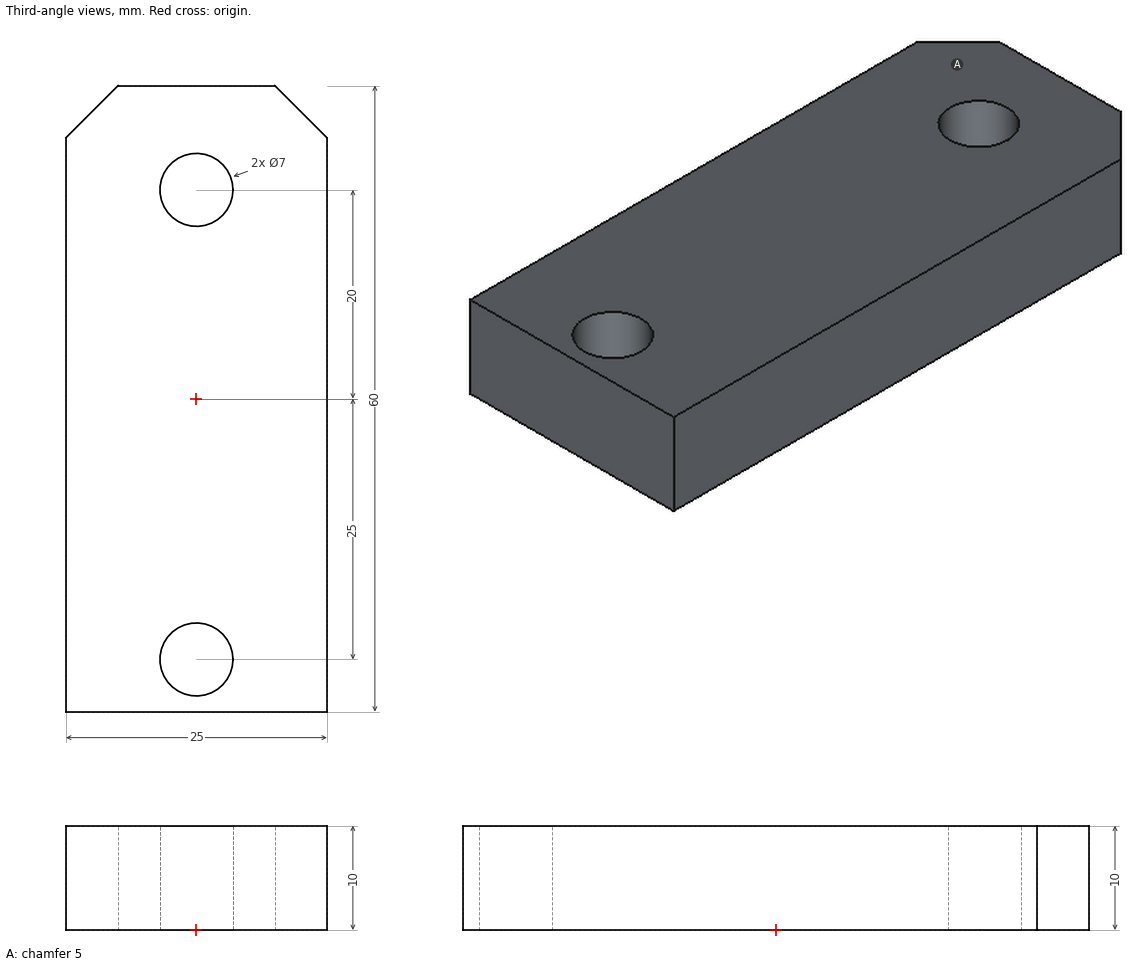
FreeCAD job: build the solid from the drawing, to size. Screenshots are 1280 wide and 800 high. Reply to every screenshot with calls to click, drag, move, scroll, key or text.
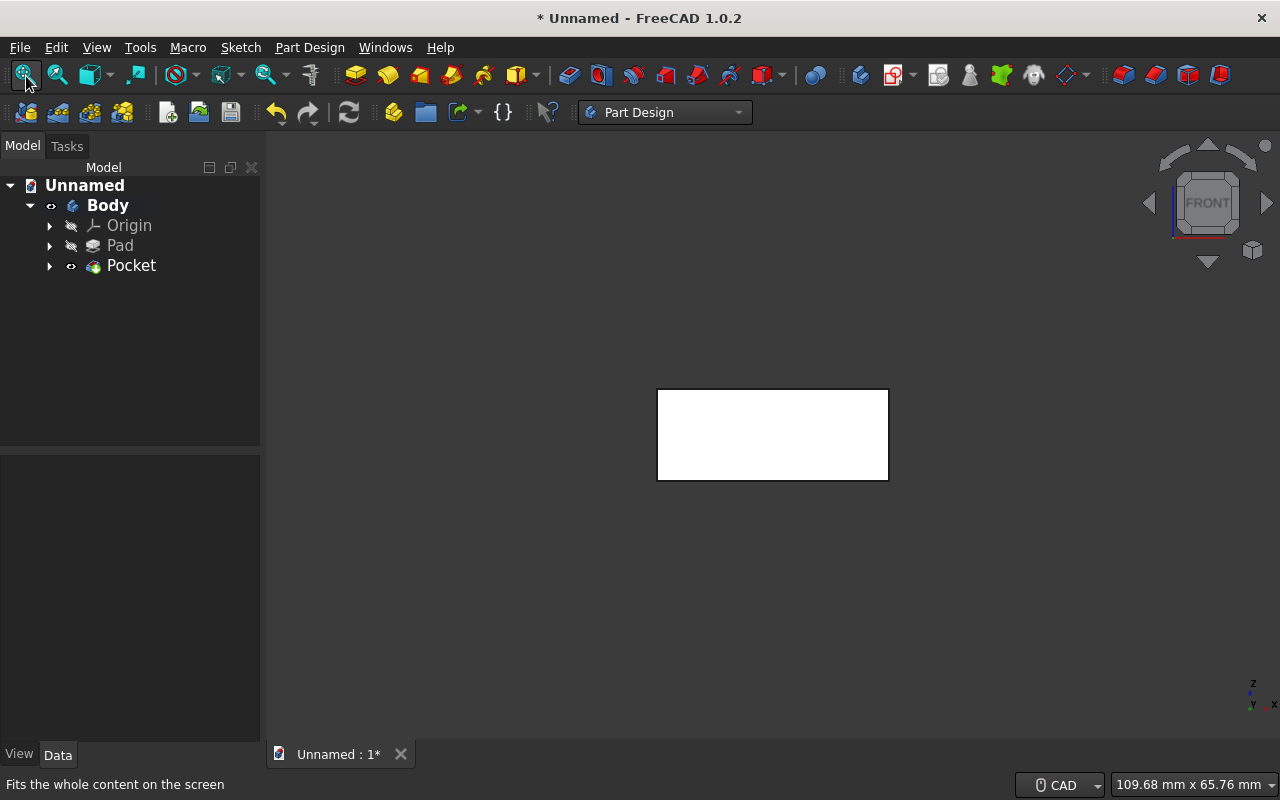
key(3)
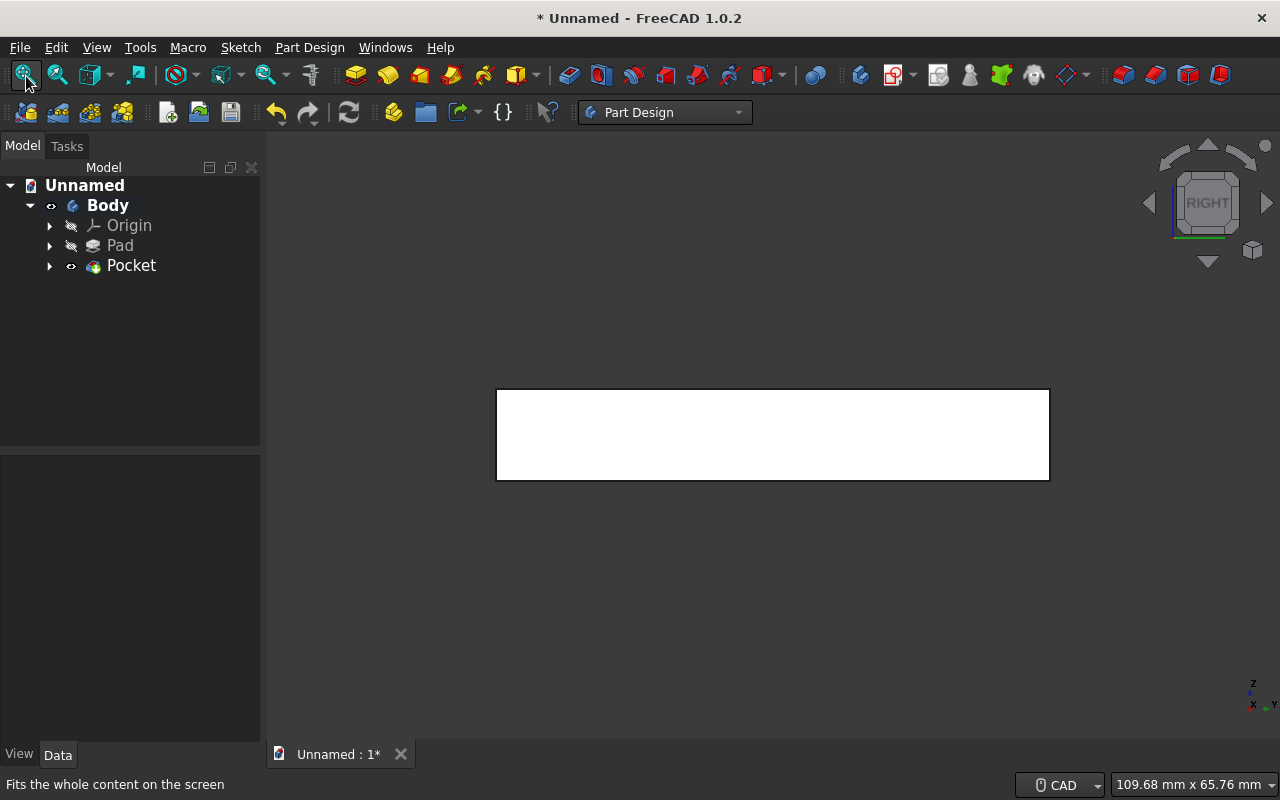
click(1050, 434)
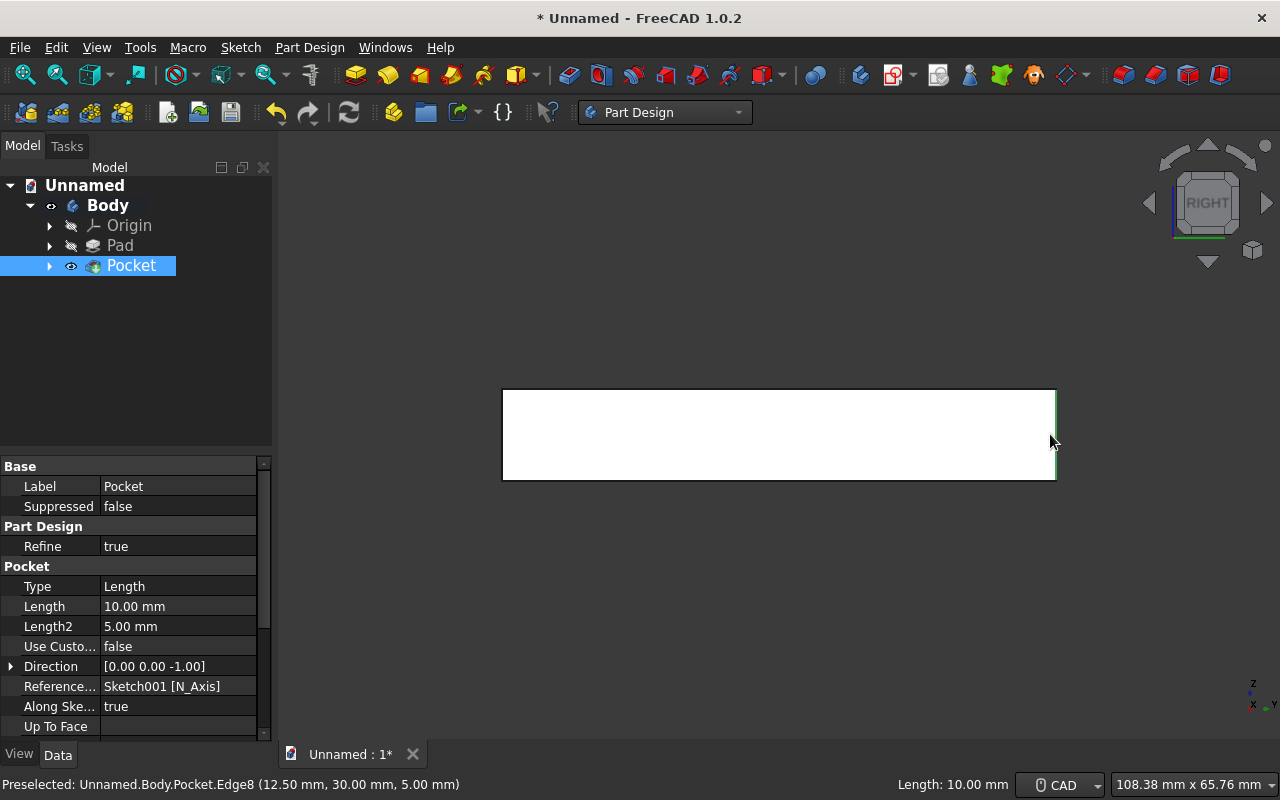
key(5)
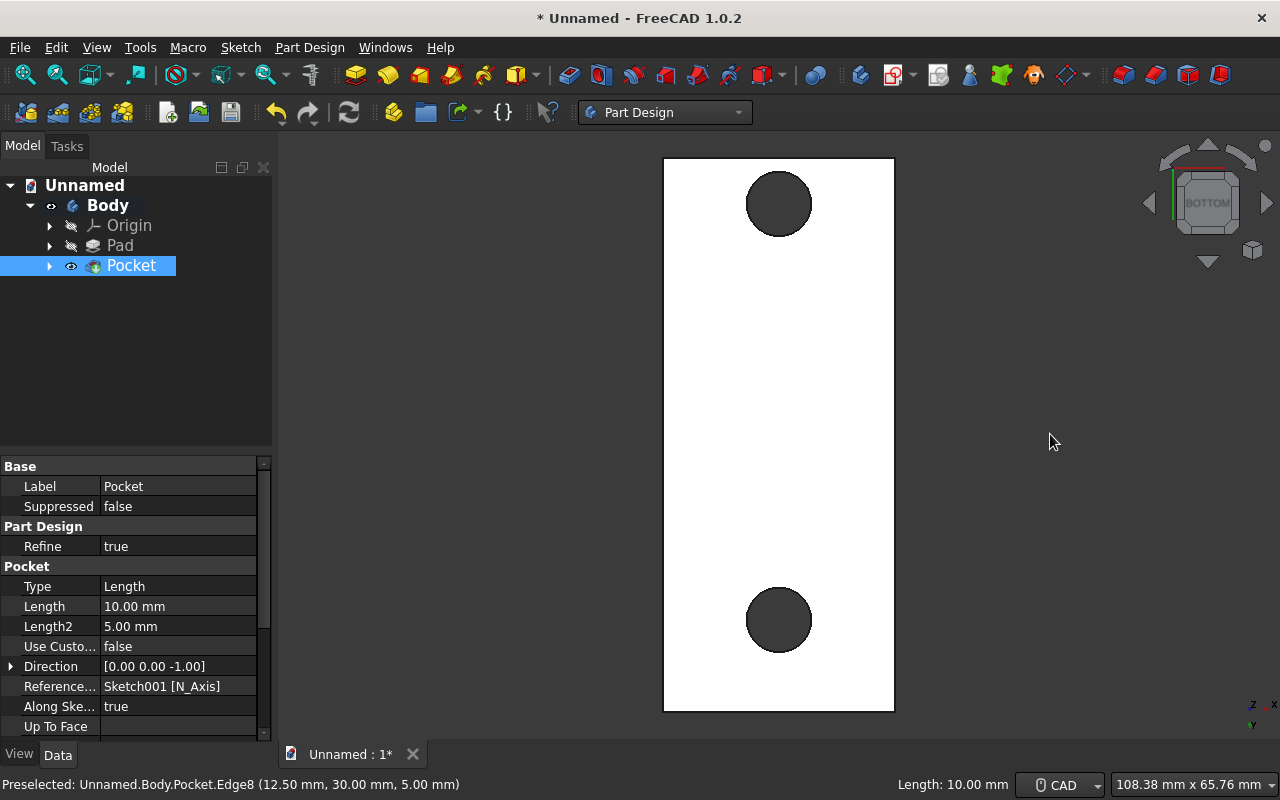
key(4)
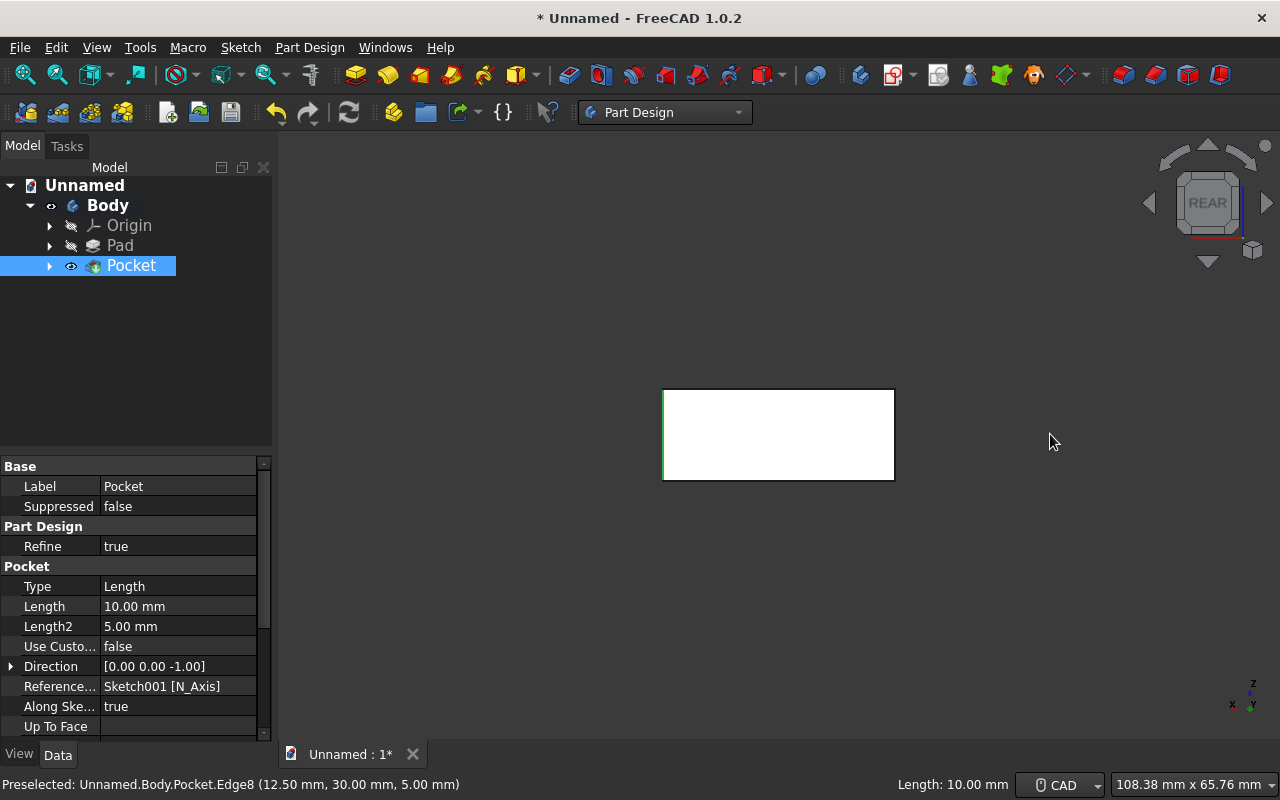
click(26, 76)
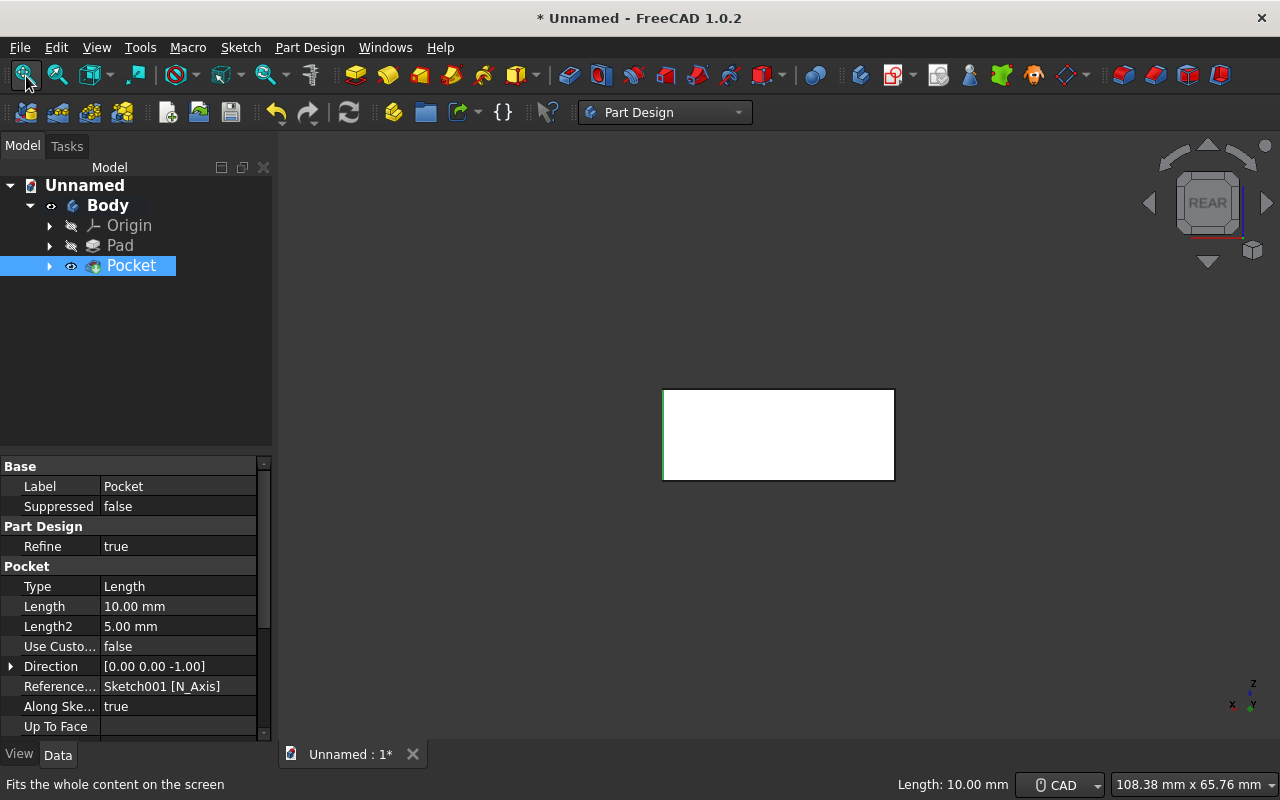
click(895, 434, ctrl)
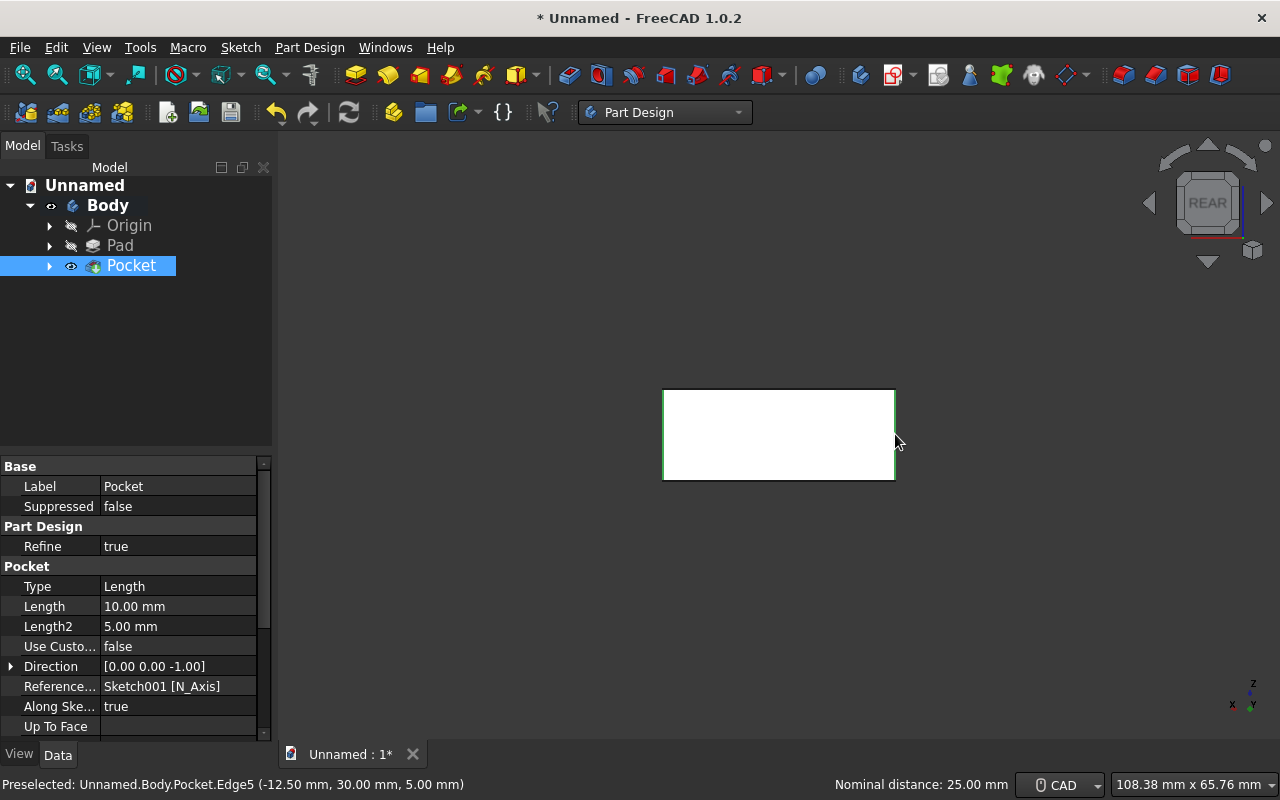
click(1156, 76)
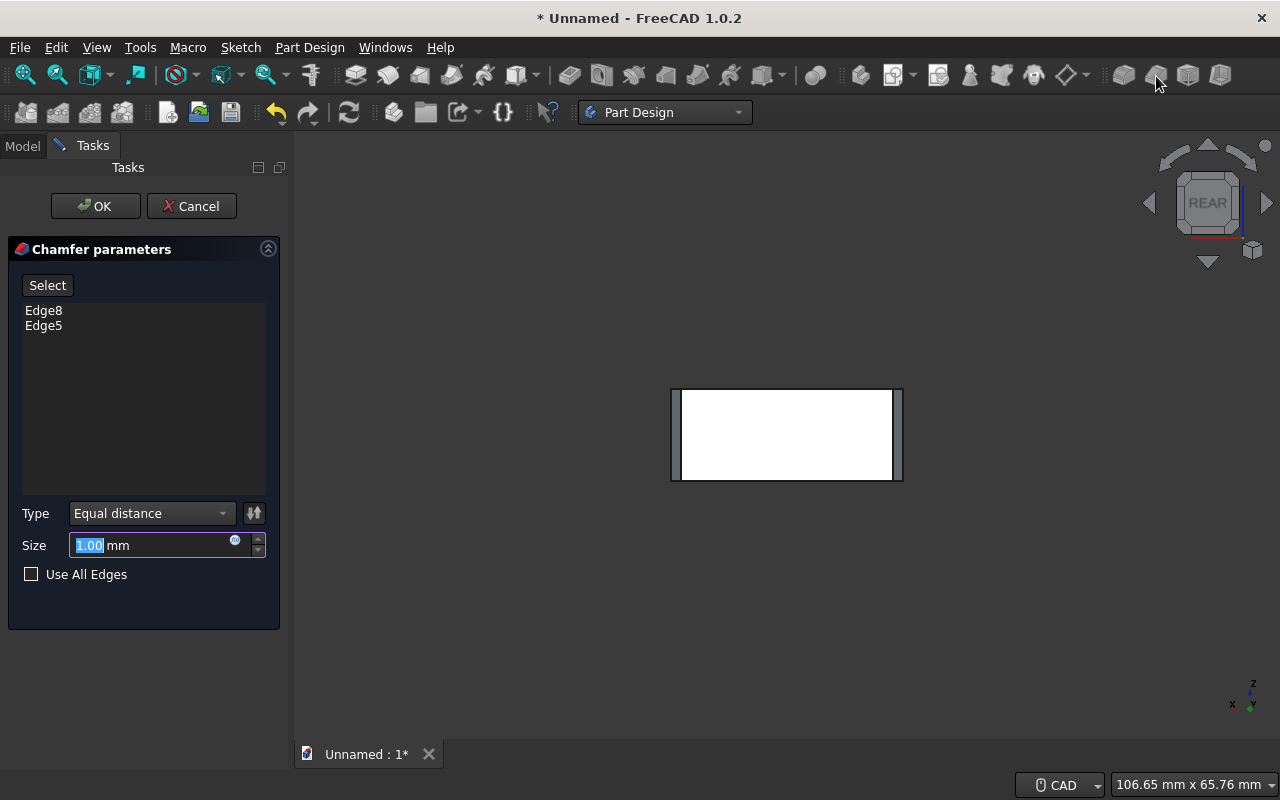
text(5)
key(Tab)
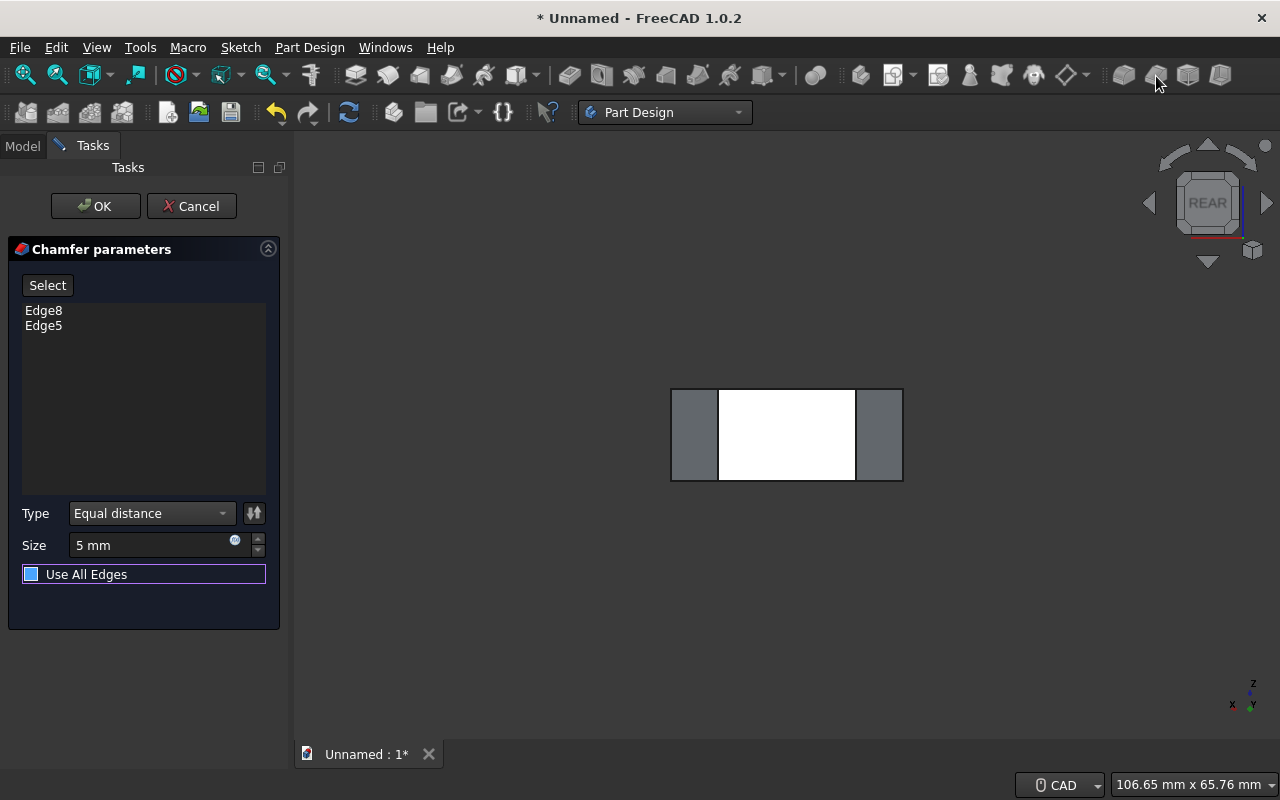
click(96, 206)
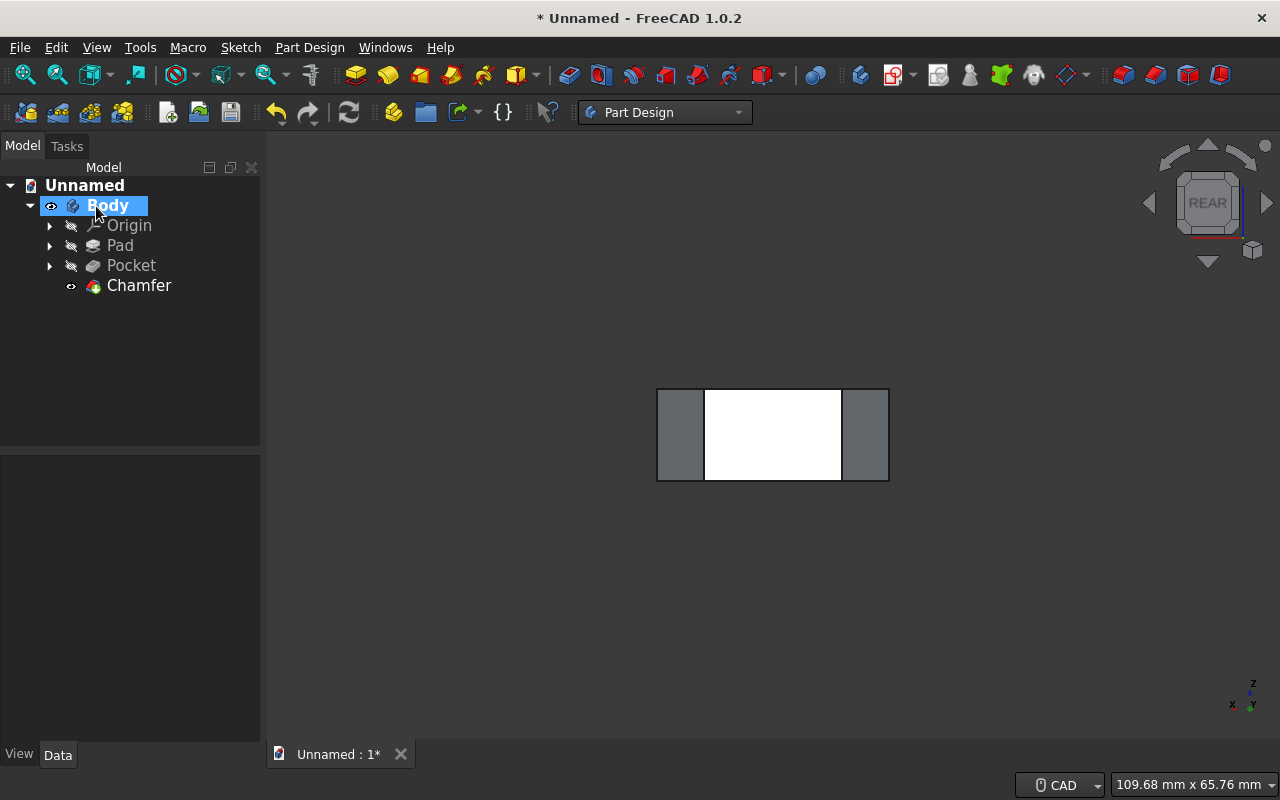
key(0)